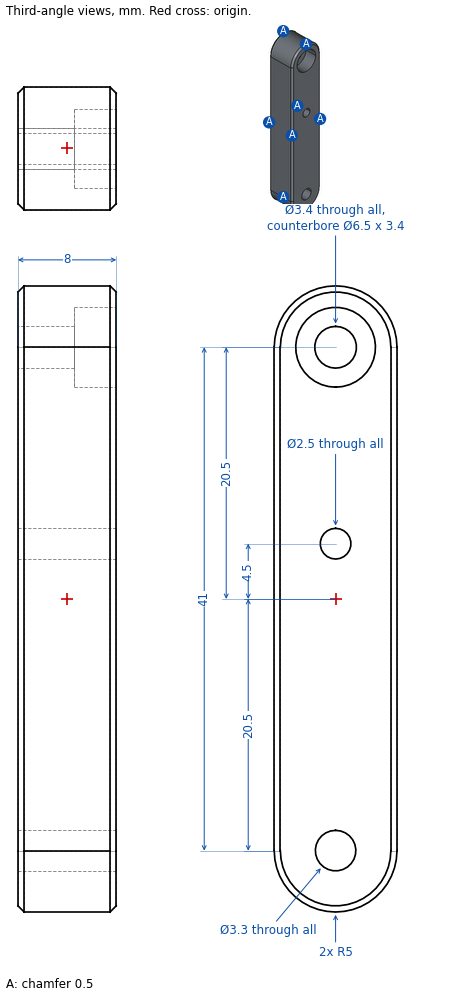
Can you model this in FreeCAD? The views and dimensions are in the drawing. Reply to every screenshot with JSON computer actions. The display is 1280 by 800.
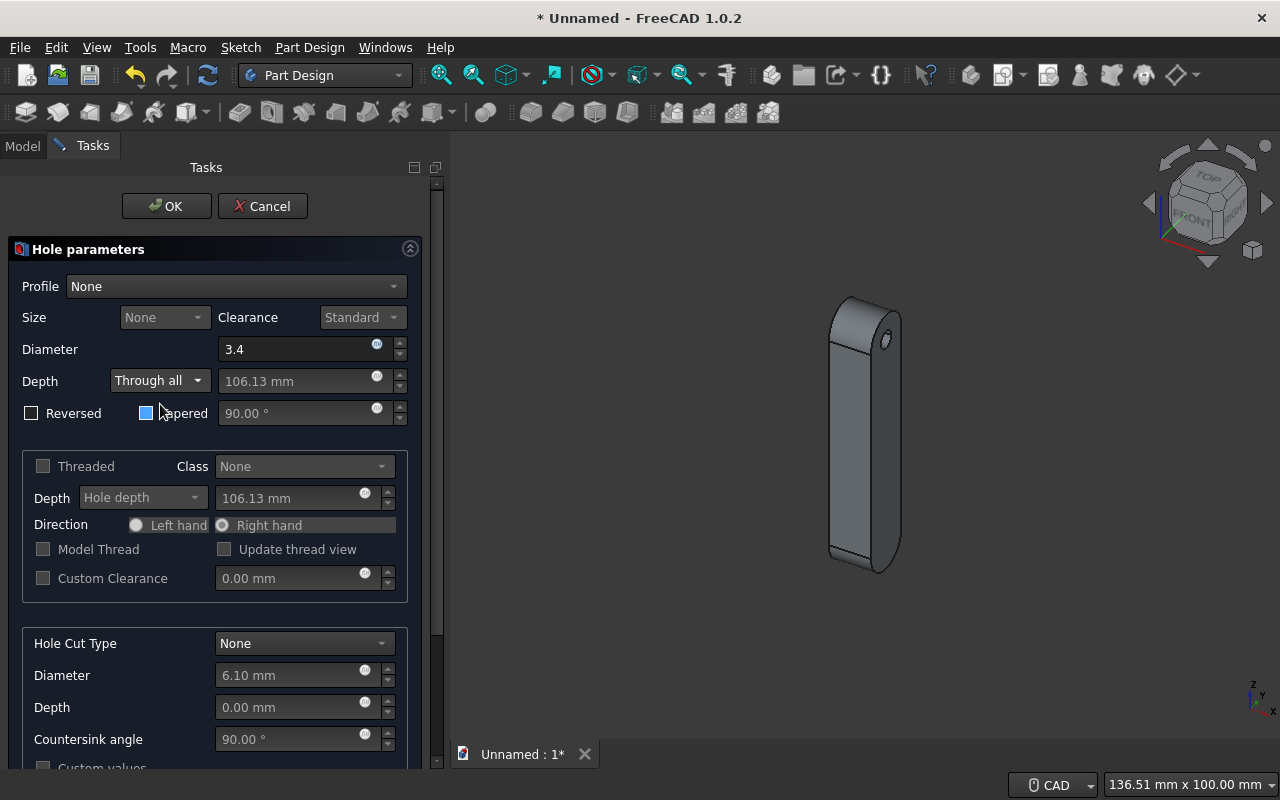
{"action": "left_click", "coordinate": [306, 644]}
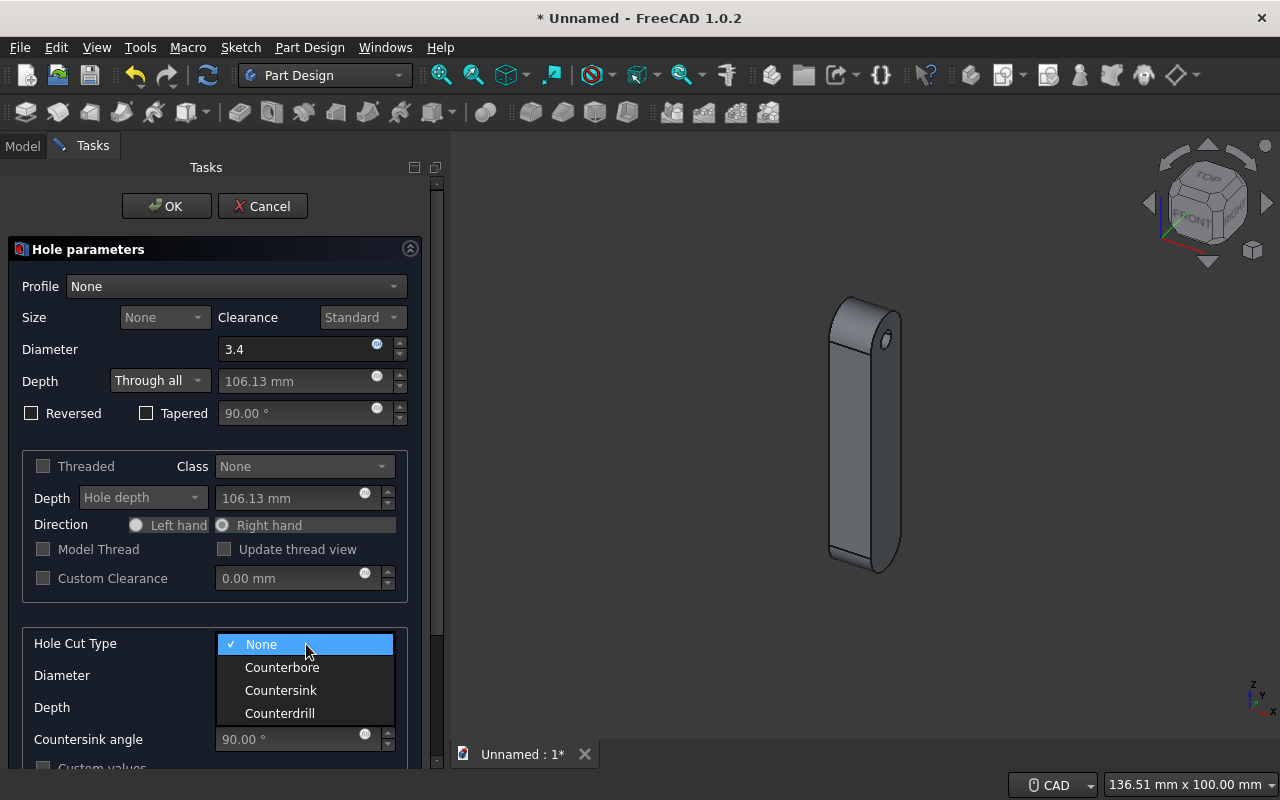
{"action": "left_click", "coordinate": [304, 668]}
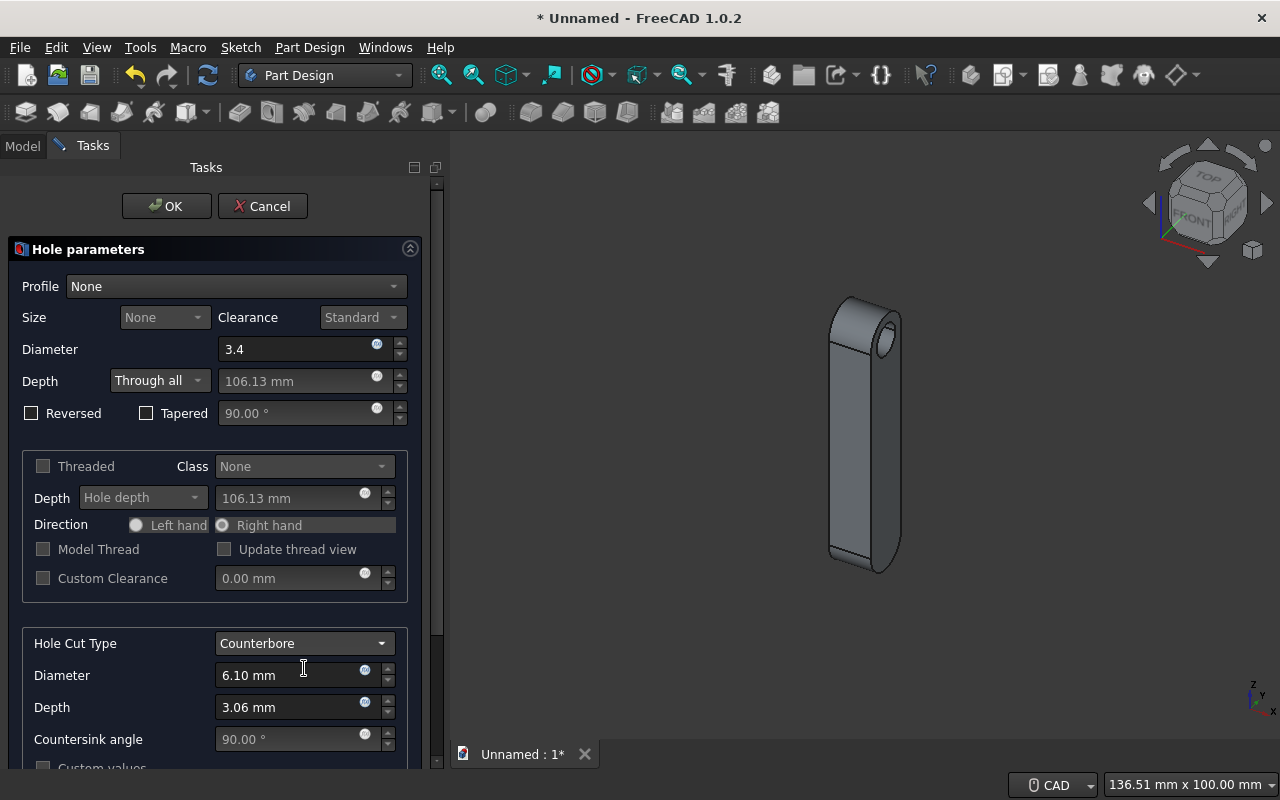
{"action": "triple_click", "coordinate": [298, 675]}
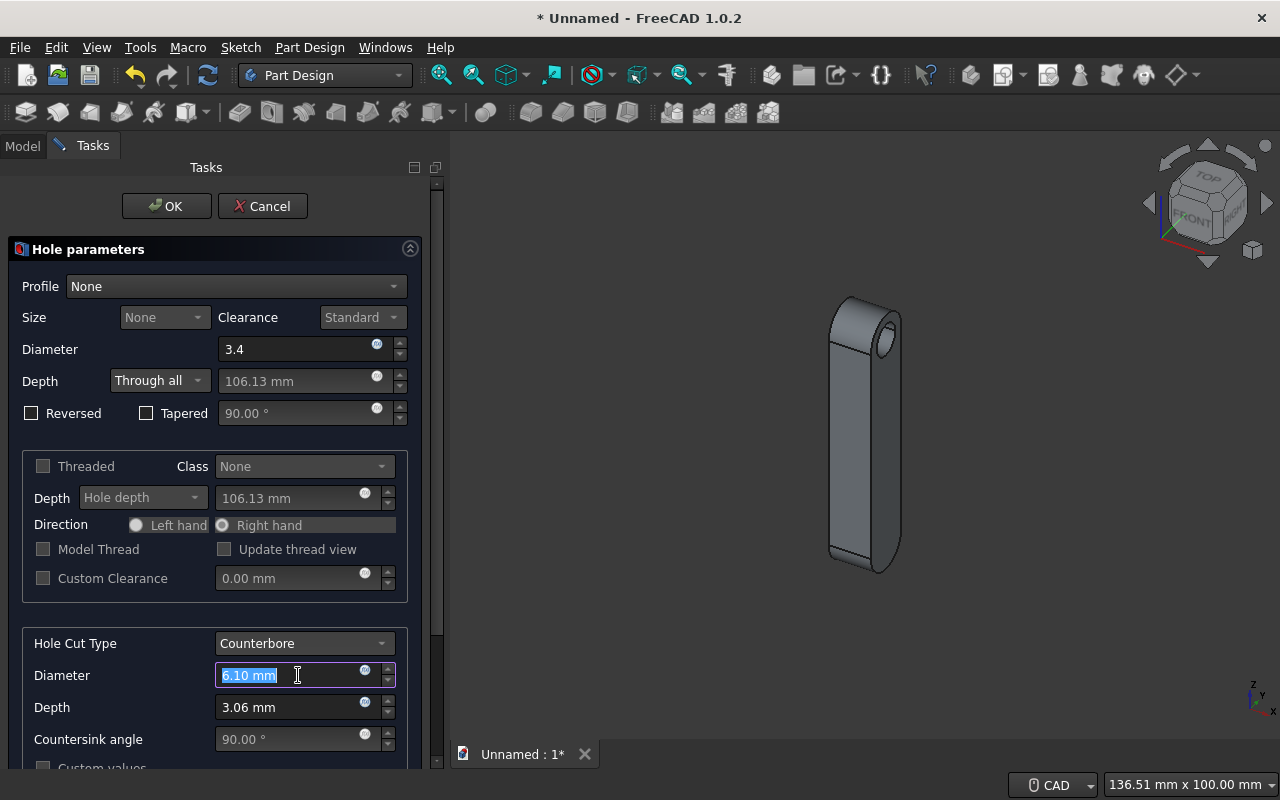
{"action": "type", "text": "6.5"}
{"action": "key", "text": "Tab"}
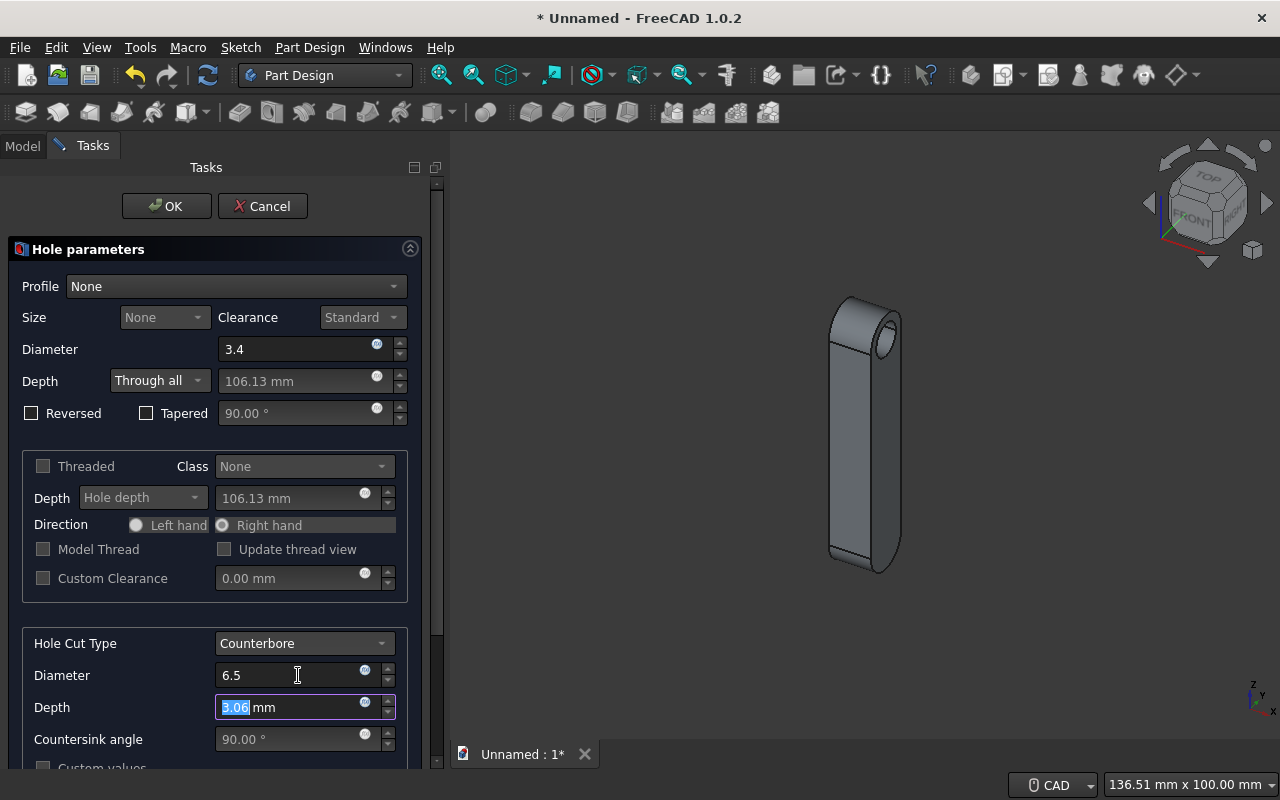
{"action": "type", "text": "3.4"}
{"action": "key", "text": "Tab"}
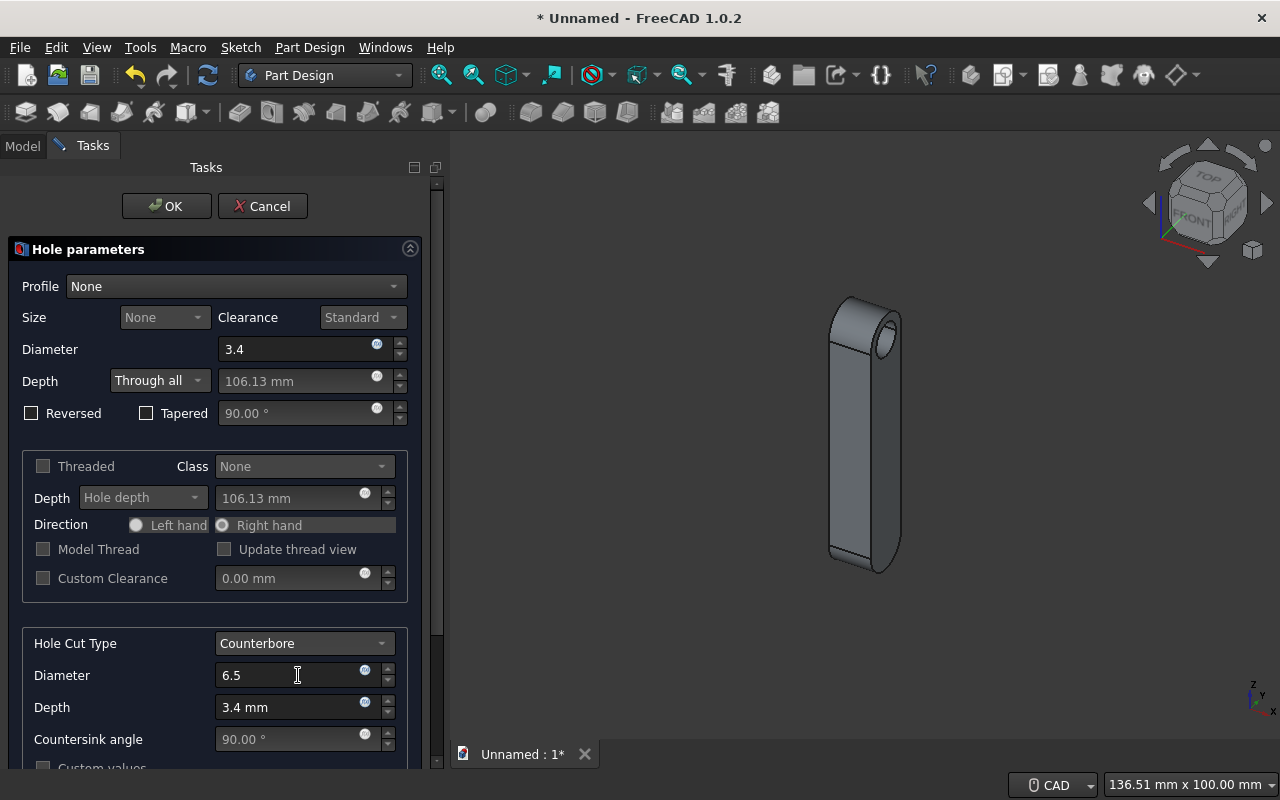
{"action": "left_click", "coordinate": [167, 206]}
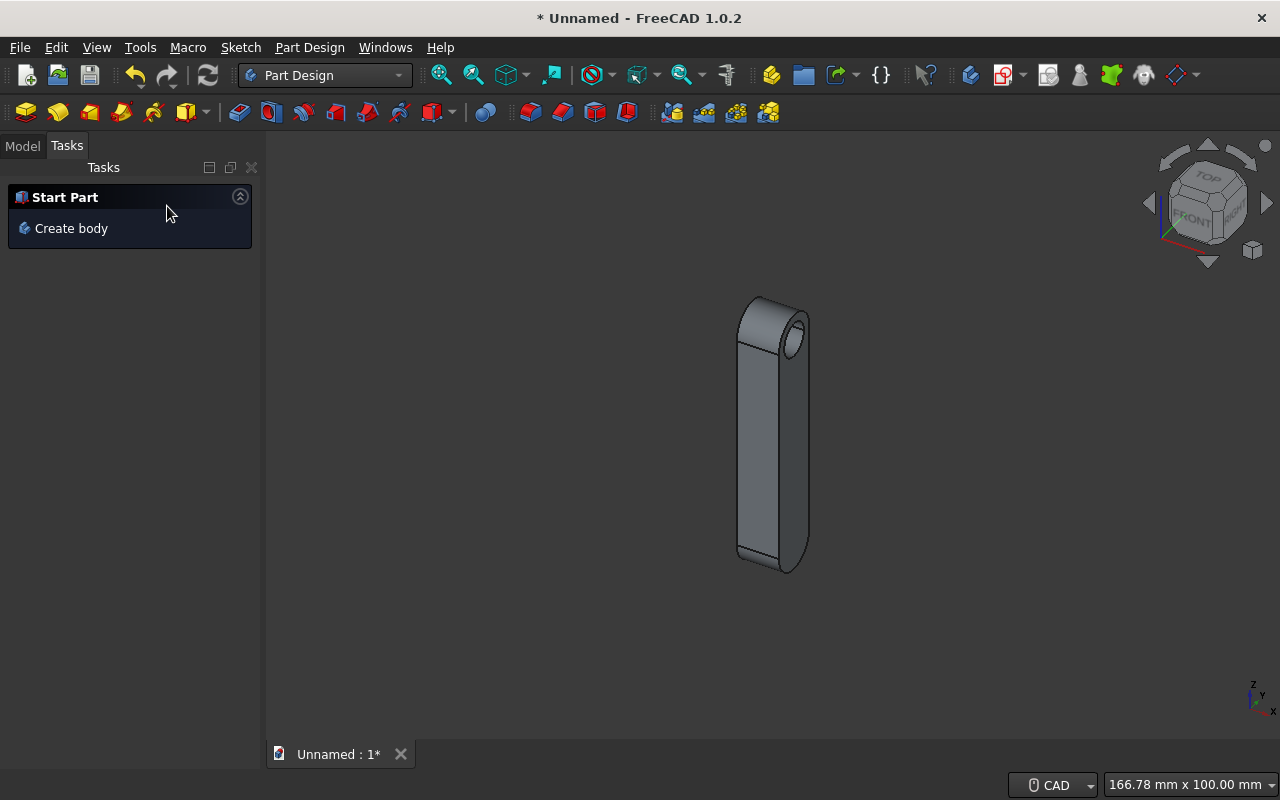
{"action": "left_click", "coordinate": [794, 514]}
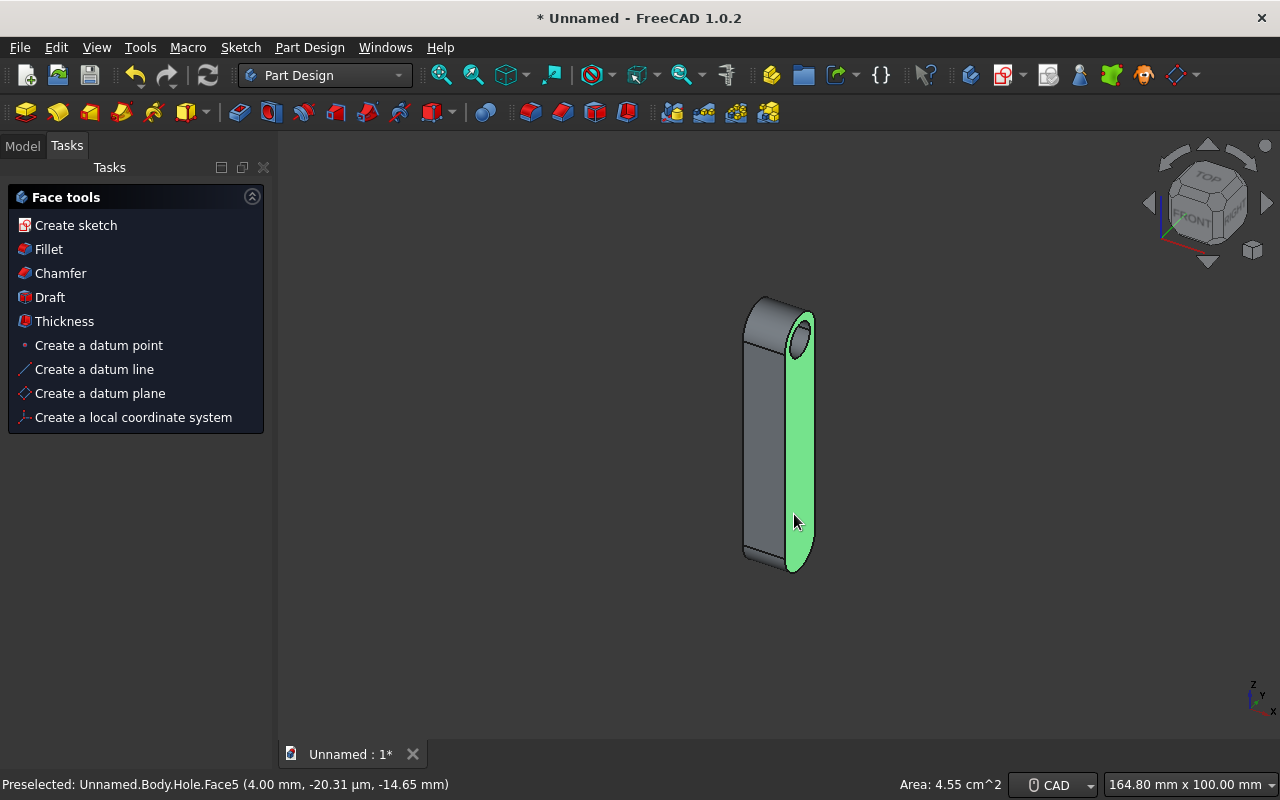
{"action": "left_click", "coordinate": [1004, 76]}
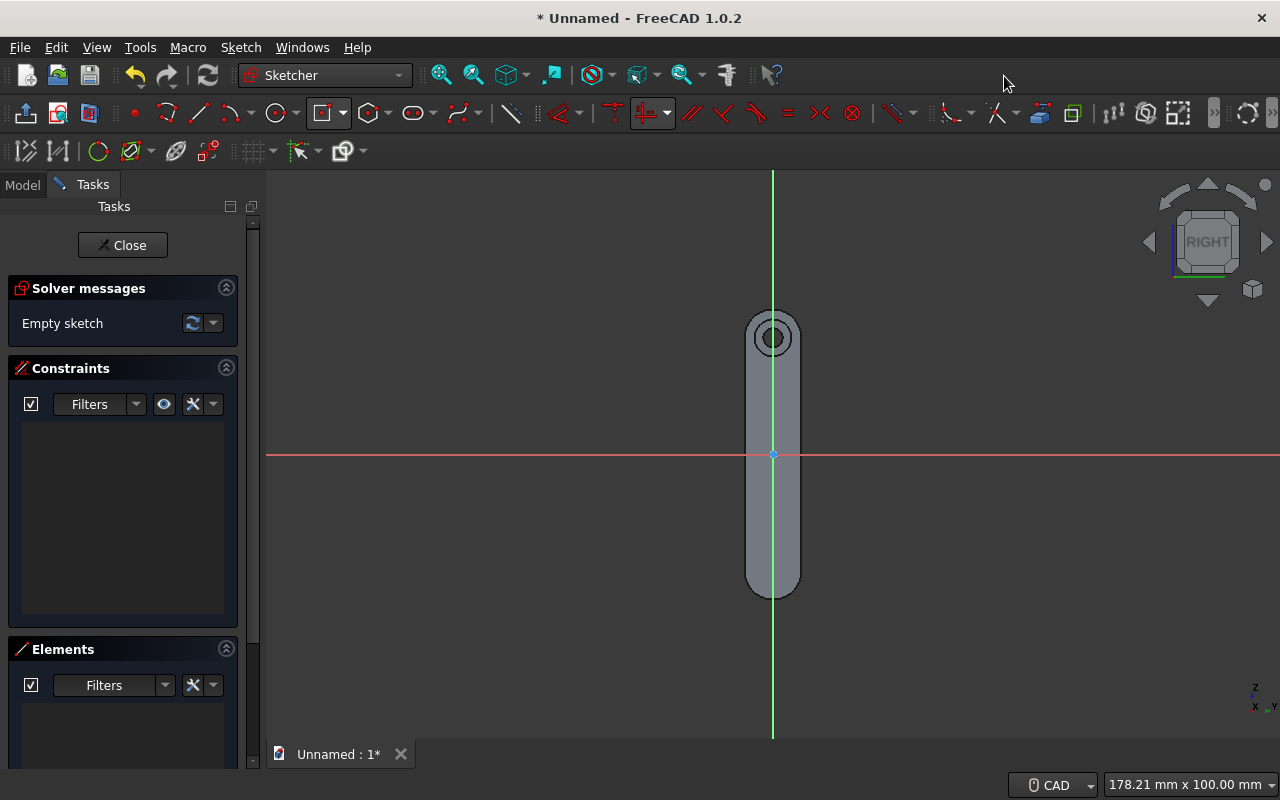
{"action": "scroll", "coordinate": [780, 437], "scroll_direction": "up", "scroll_amount": 12}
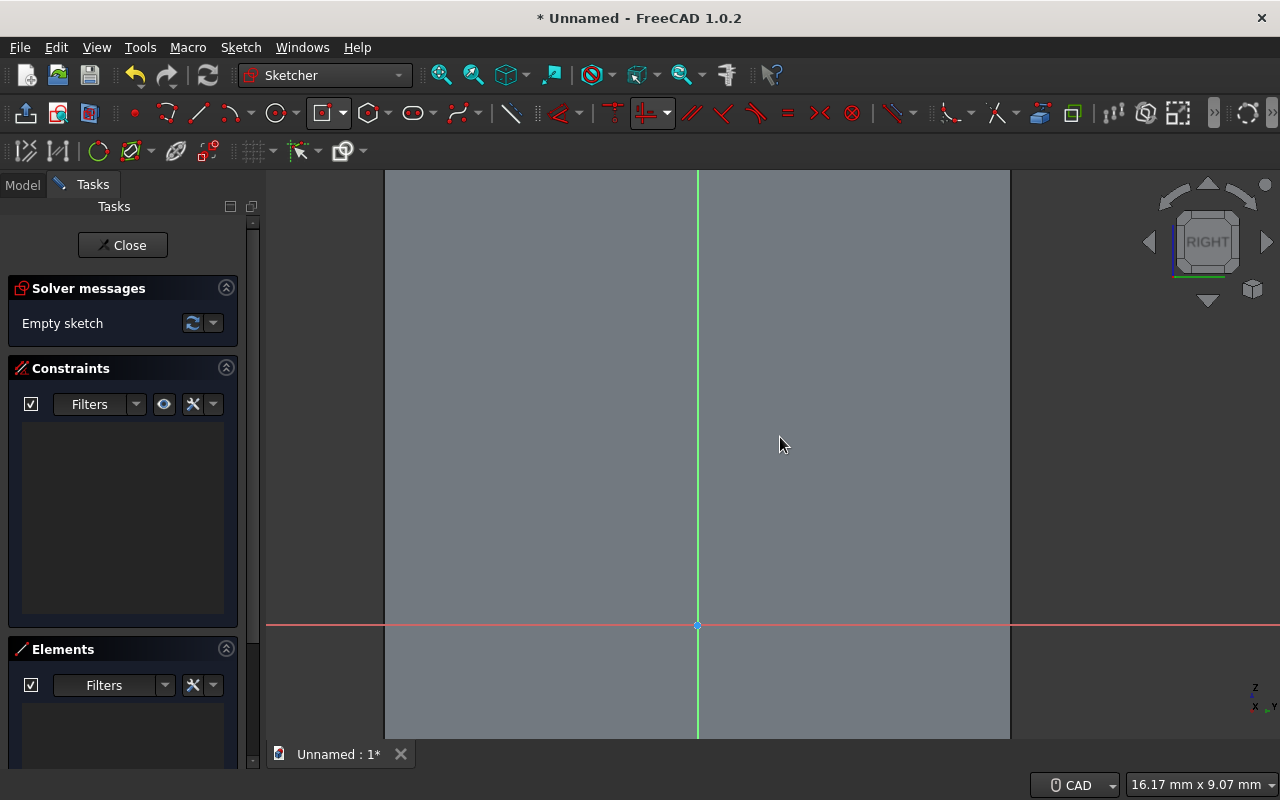
{"action": "left_click", "coordinate": [276, 114]}